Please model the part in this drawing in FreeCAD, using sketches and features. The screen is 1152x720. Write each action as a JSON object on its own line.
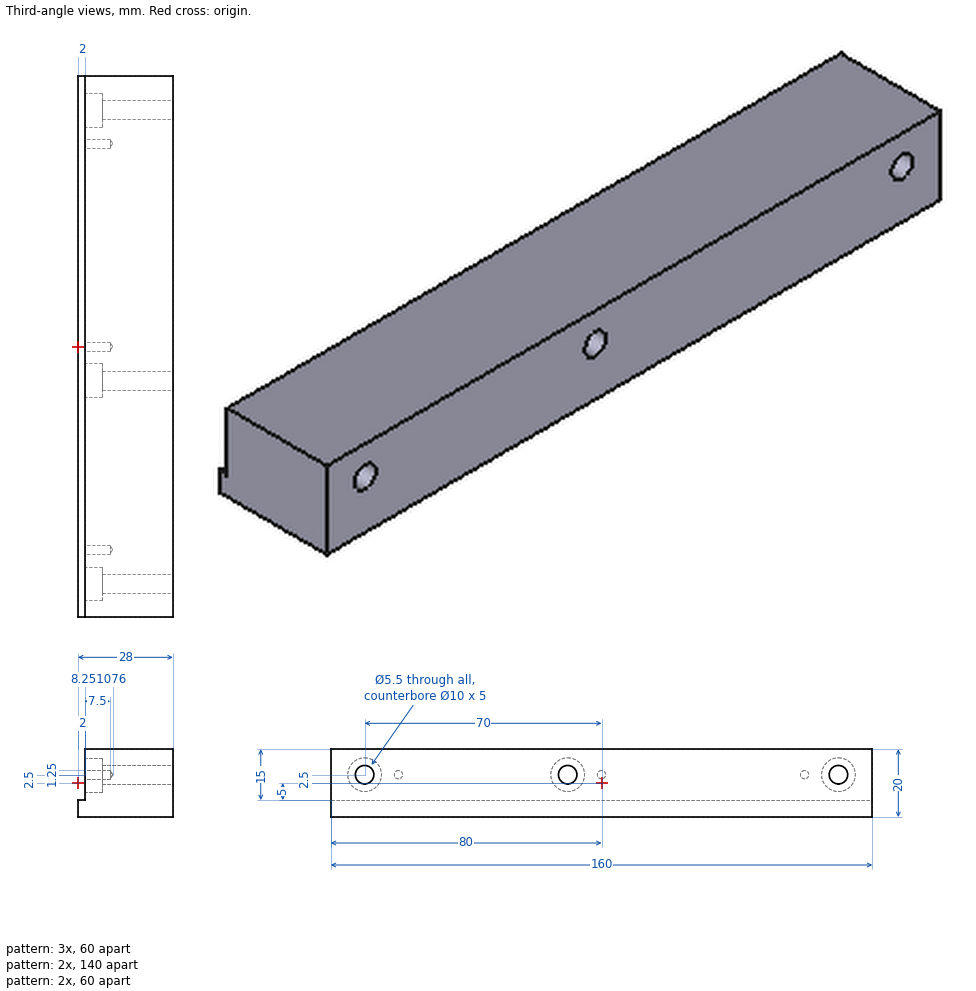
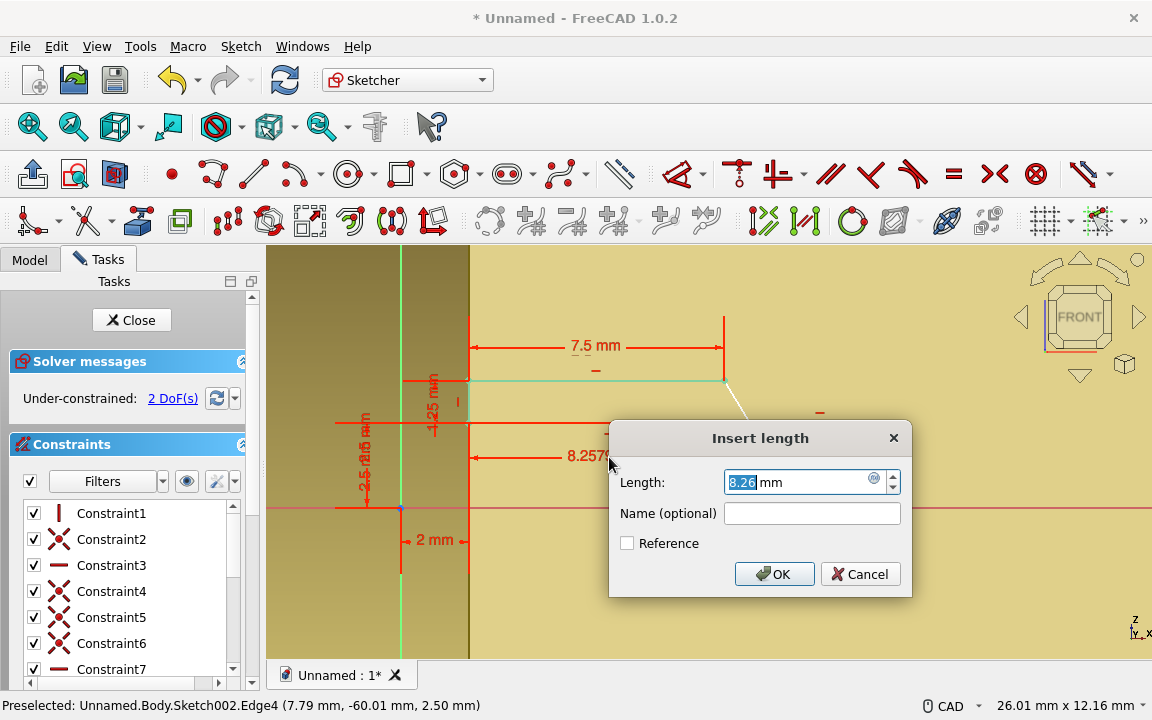
{"action": "type", "text": "8.251076"}
{"action": "key", "text": "Return"}
{"action": "key", "text": "Escape"}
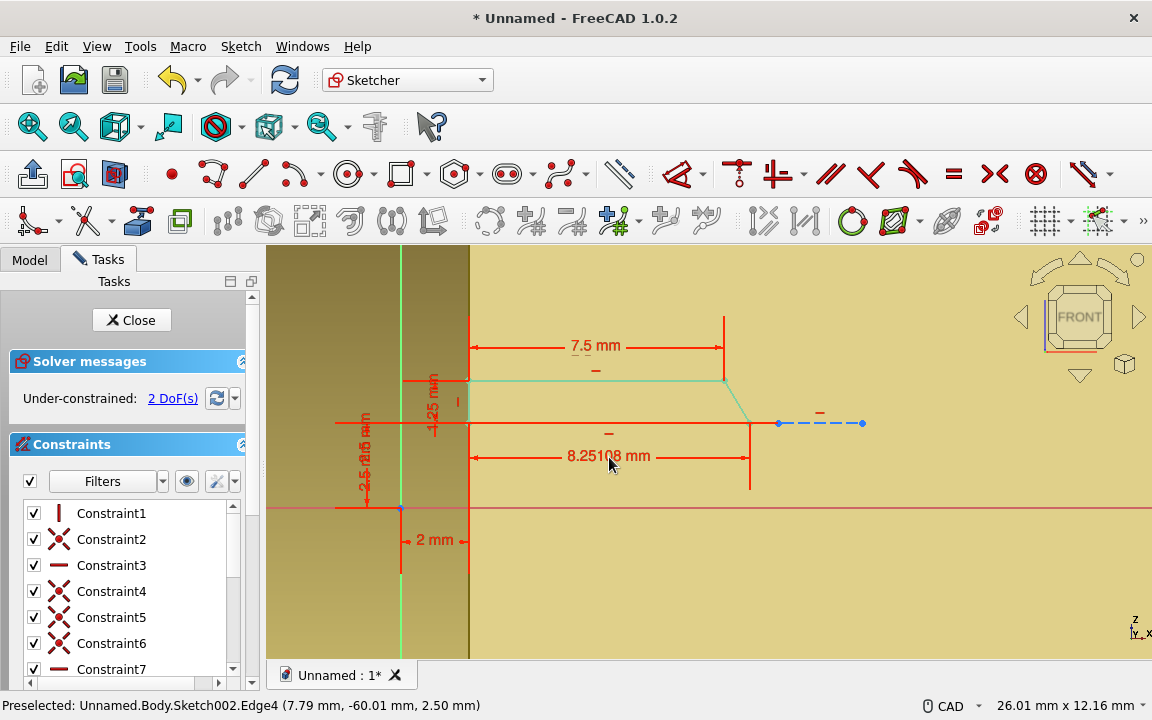
{"action": "left_click", "coordinate": [132, 320]}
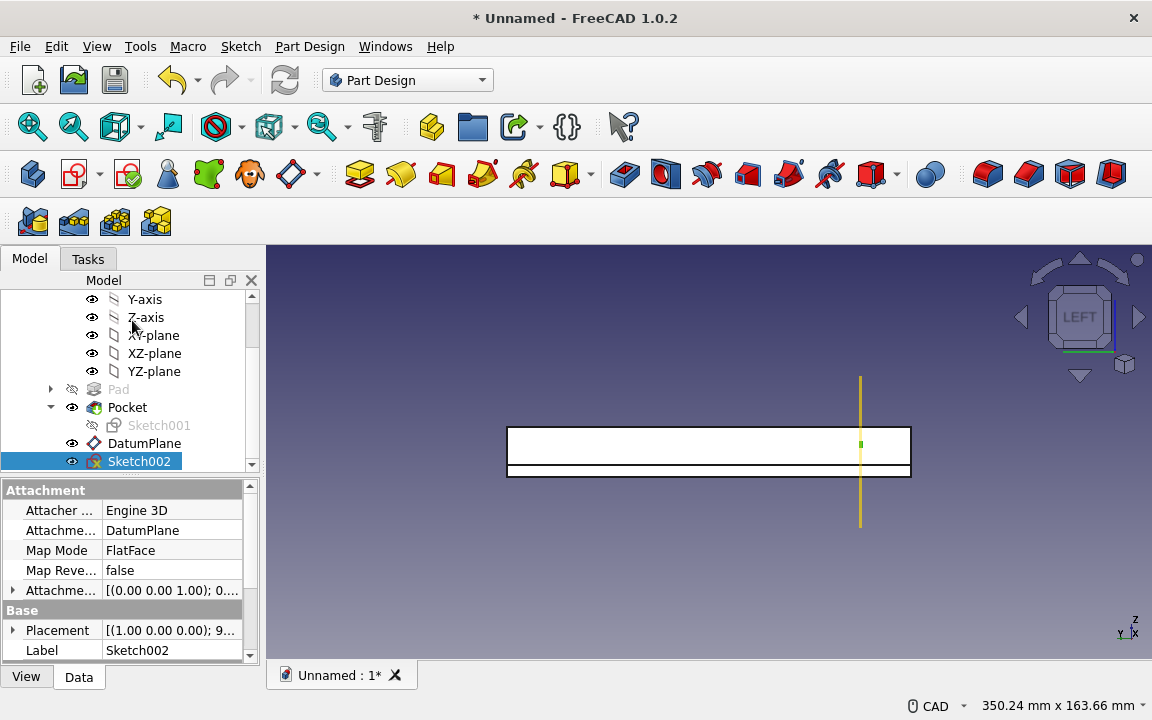
{"action": "left_click", "coordinate": [707, 174]}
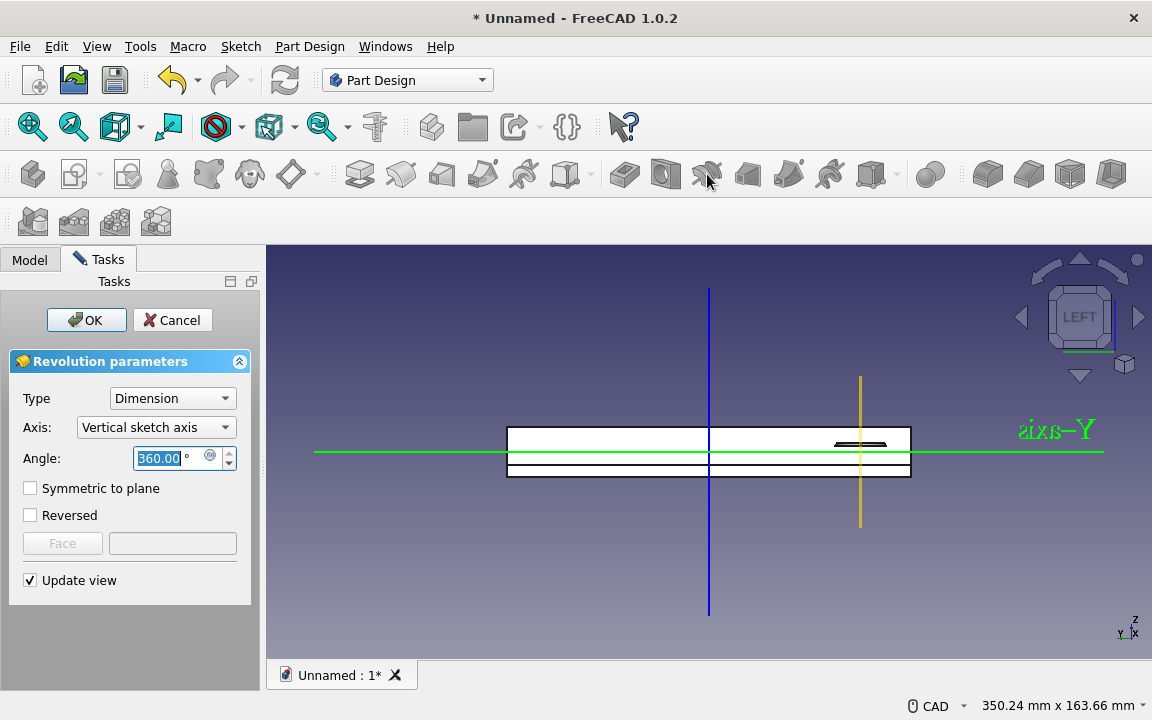
{"action": "left_click", "coordinate": [157, 428]}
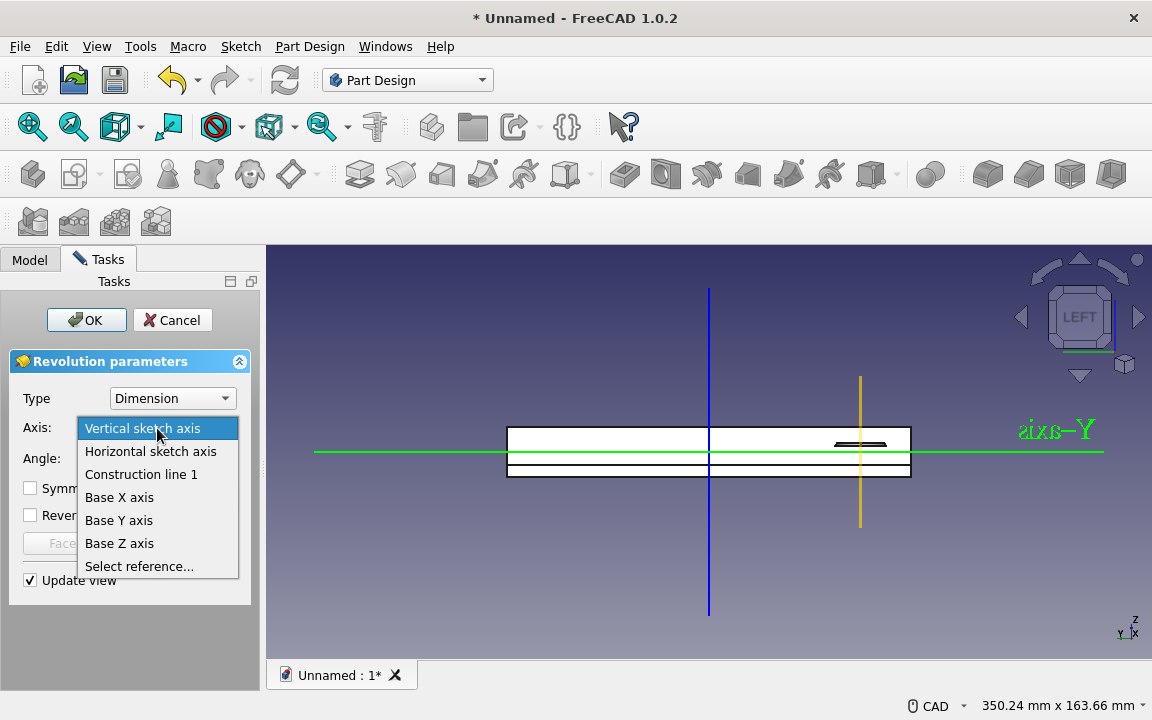
{"action": "left_click", "coordinate": [156, 474]}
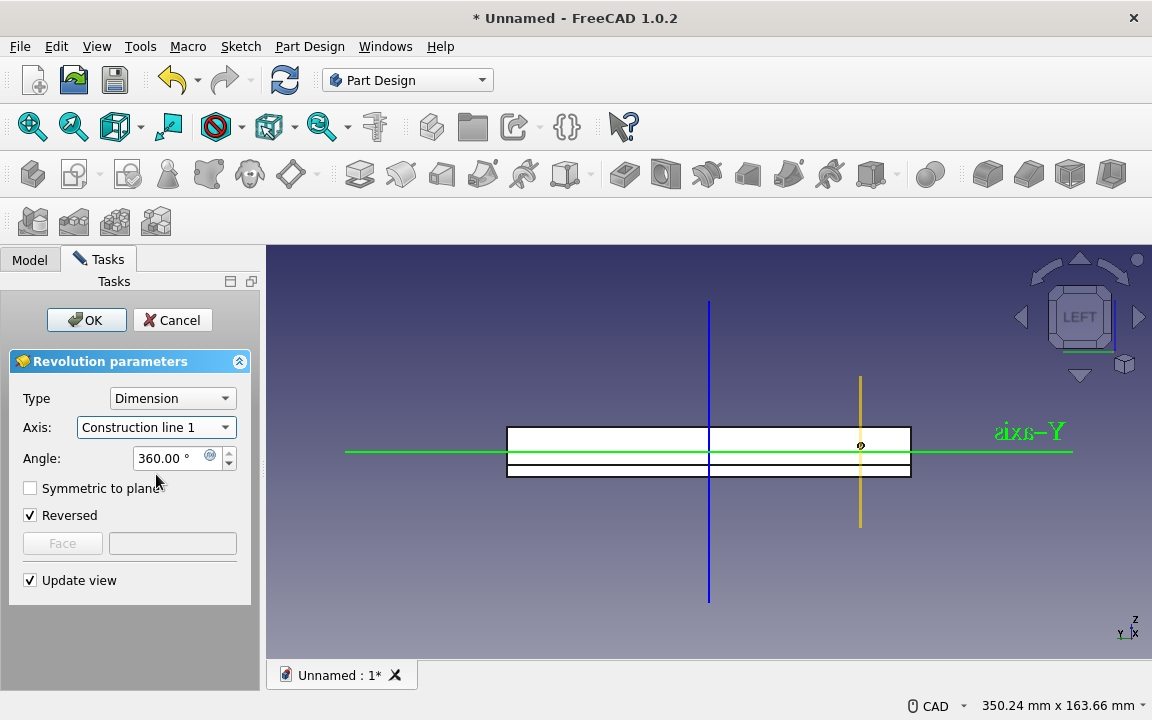
{"action": "left_click", "coordinate": [87, 320]}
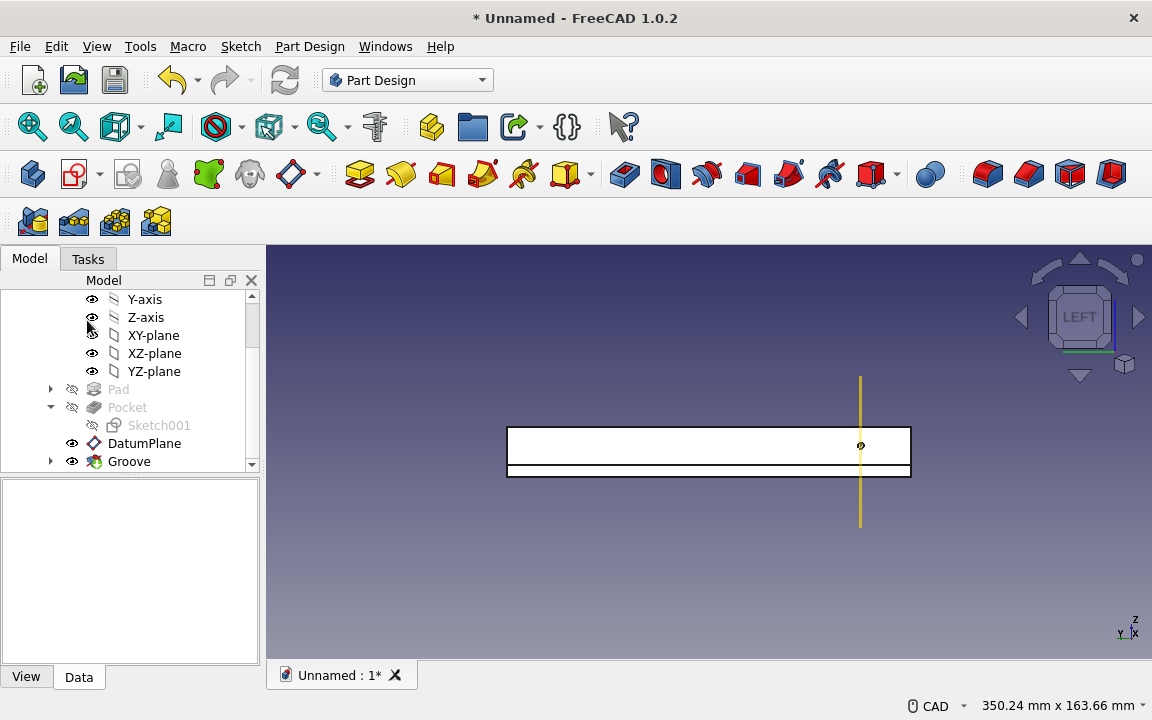
{"action": "left_click", "coordinate": [117, 443]}
{"action": "key", "text": "space"}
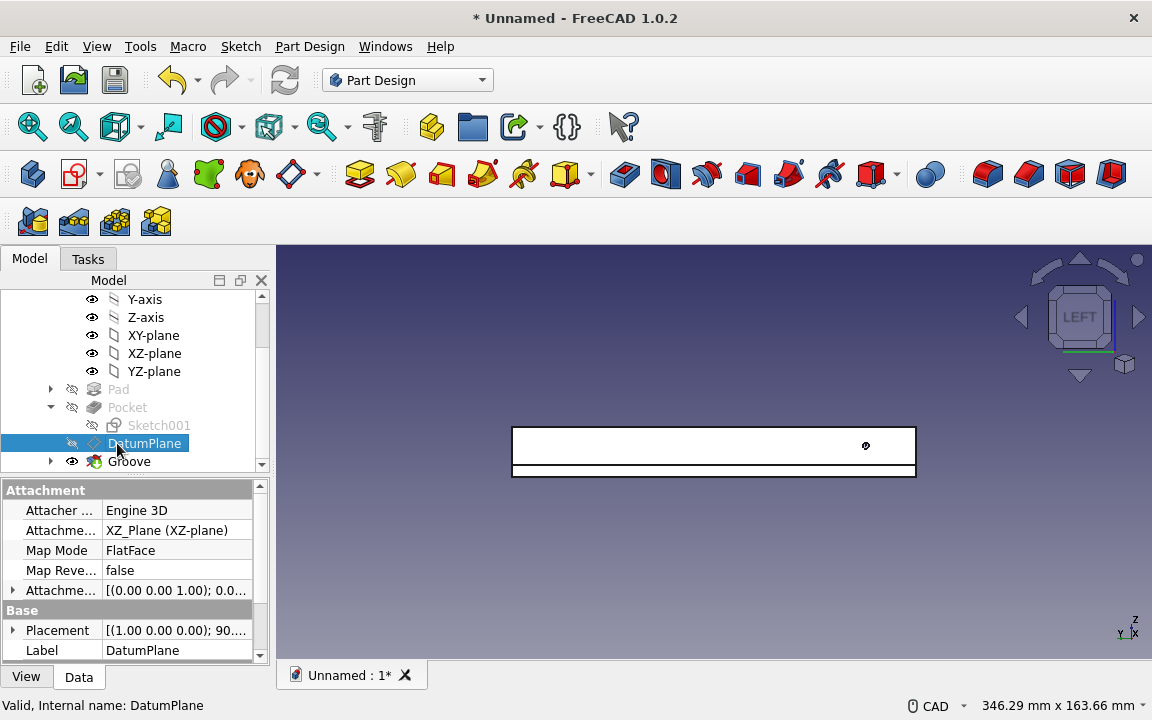
{"action": "left_click", "coordinate": [117, 461]}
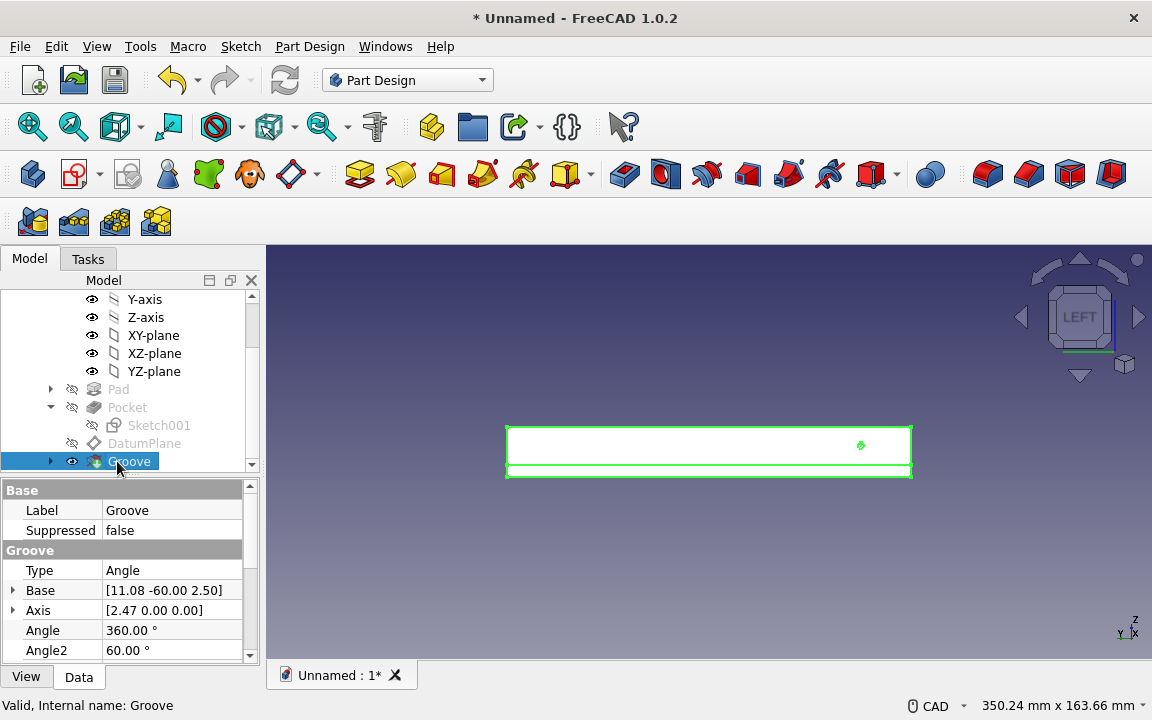
{"action": "left_click", "coordinate": [74, 222]}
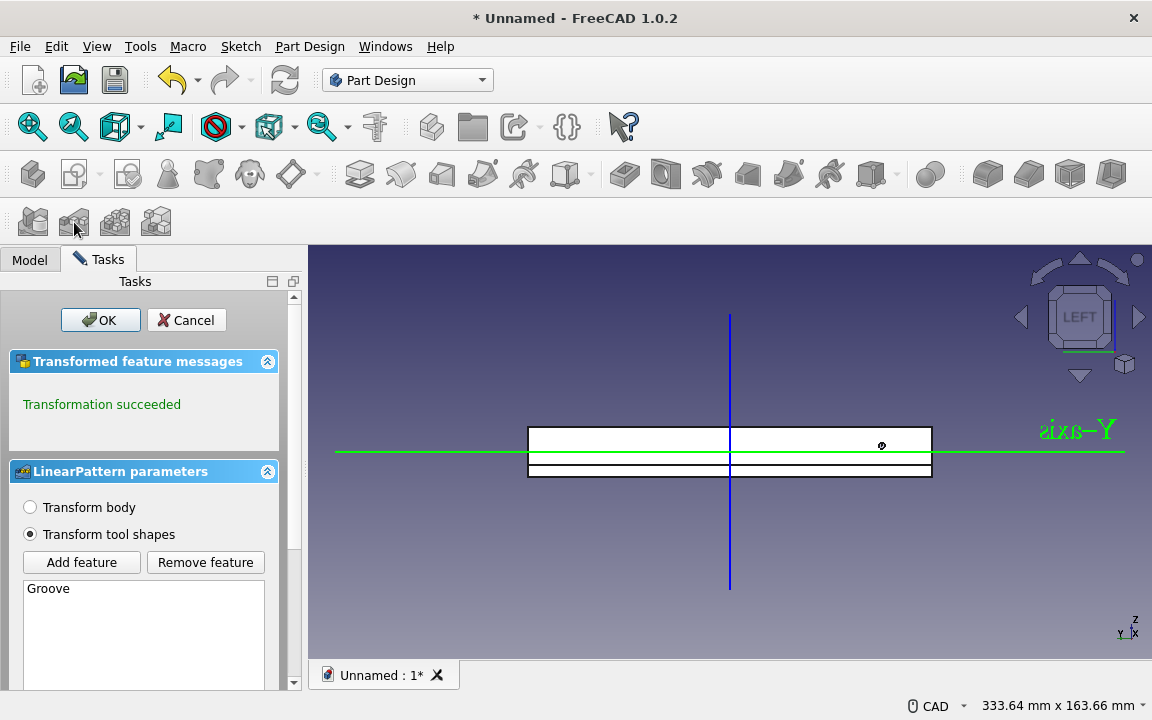
{"action": "scroll", "coordinate": [294, 490], "scroll_direction": "down", "scroll_amount": 2}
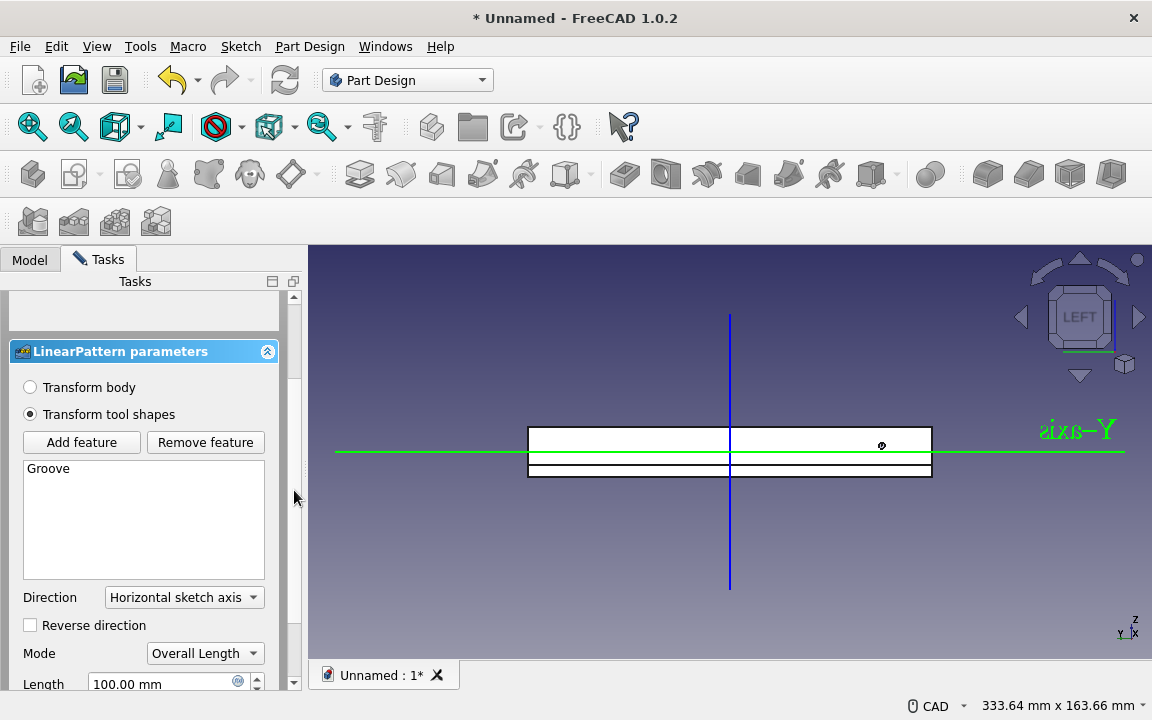
{"action": "left_click", "coordinate": [185, 598]}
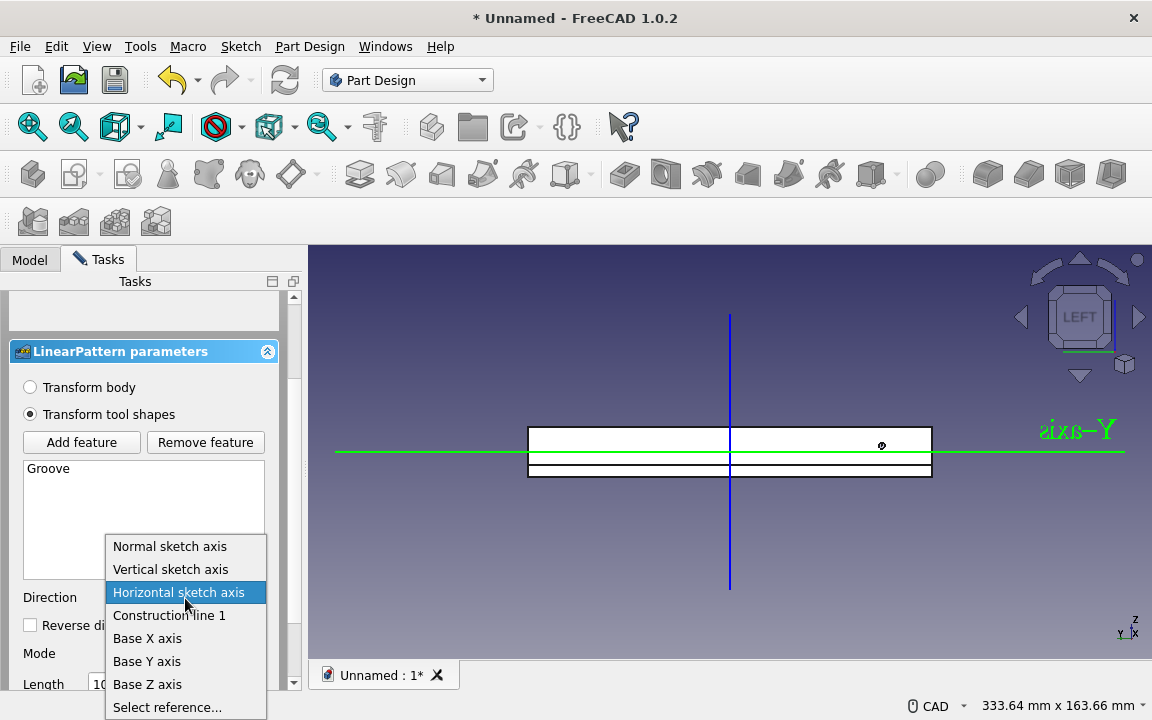
{"action": "left_click", "coordinate": [184, 662]}